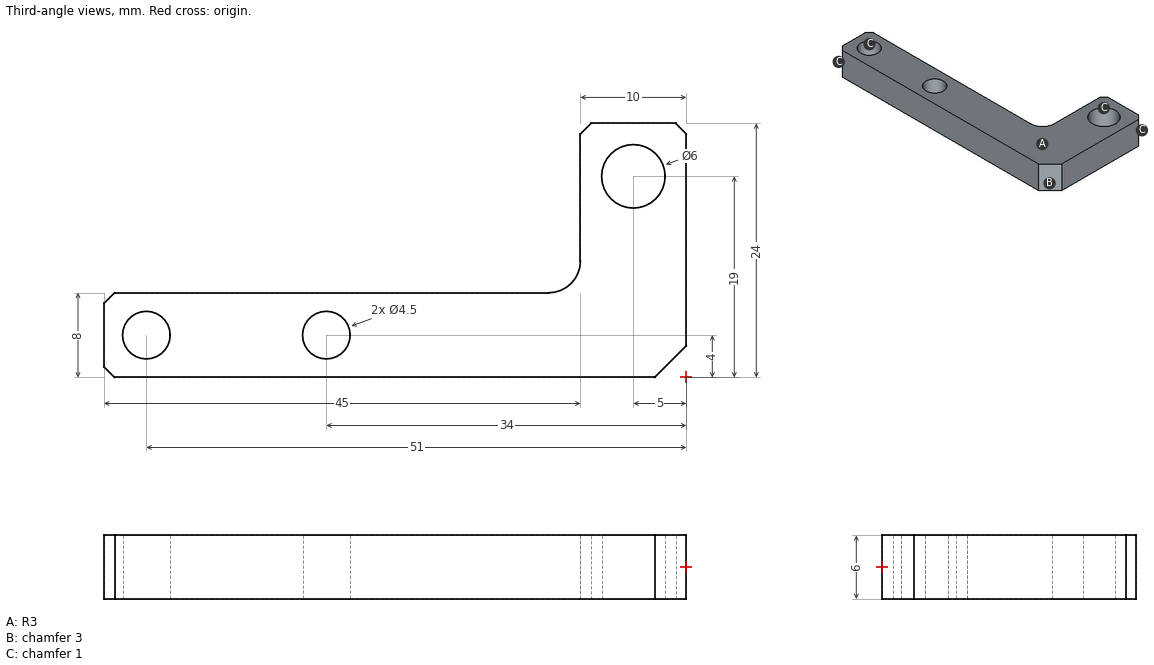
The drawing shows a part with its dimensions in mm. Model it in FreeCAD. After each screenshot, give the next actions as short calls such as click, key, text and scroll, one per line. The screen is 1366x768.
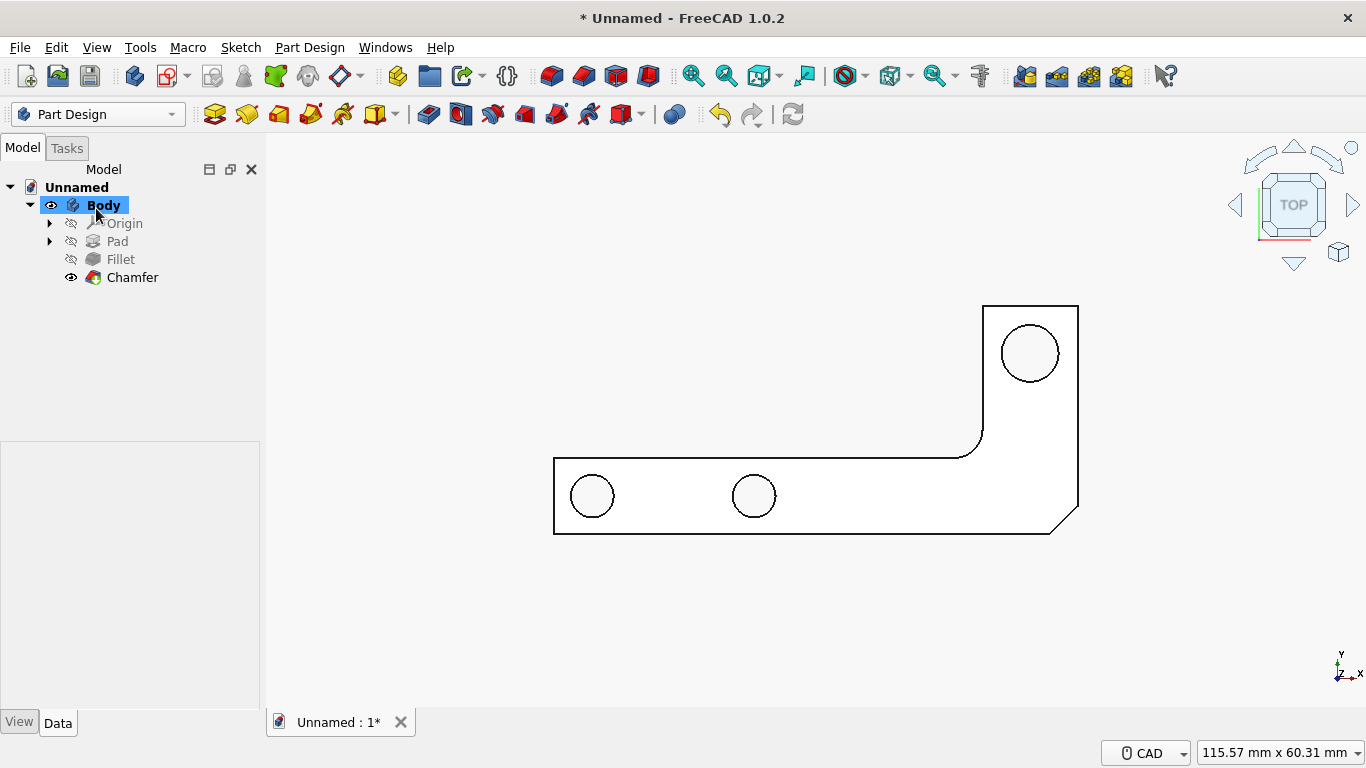
key(0)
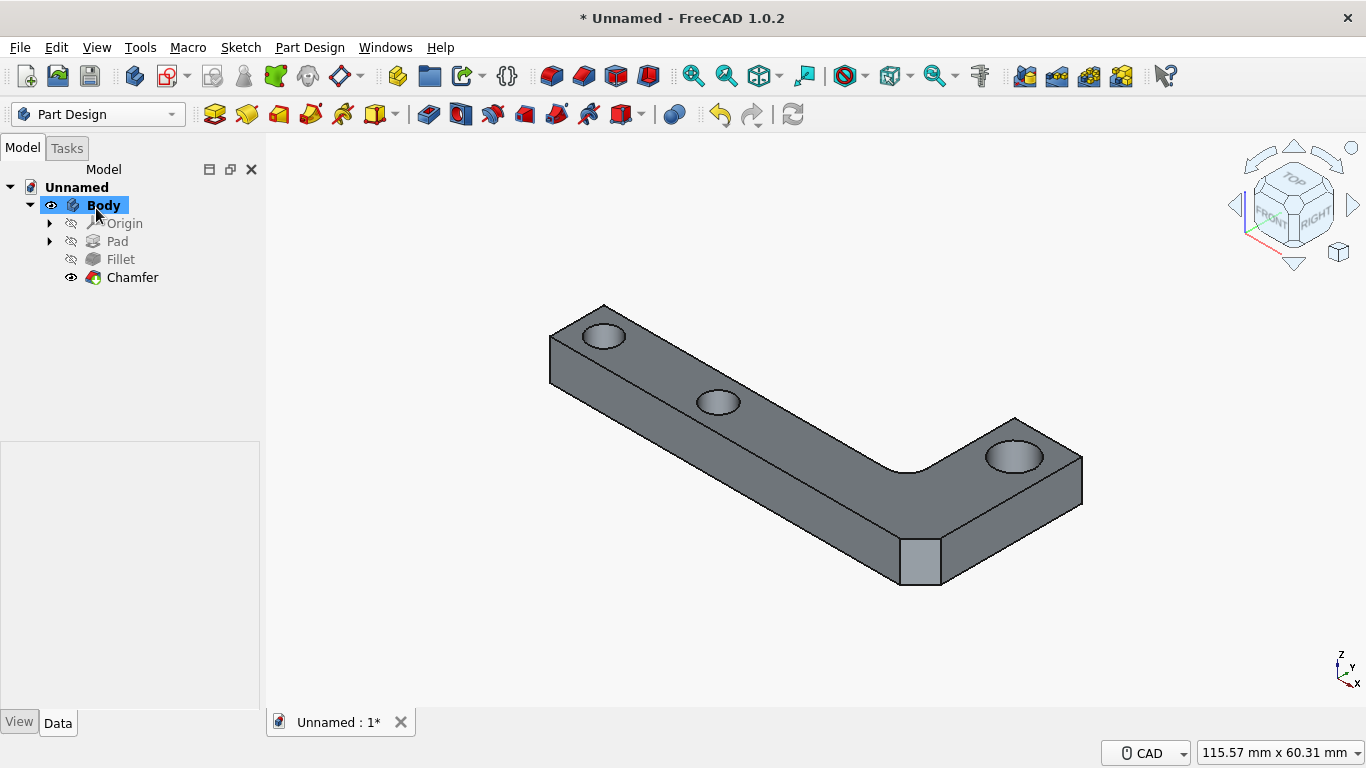
key(1)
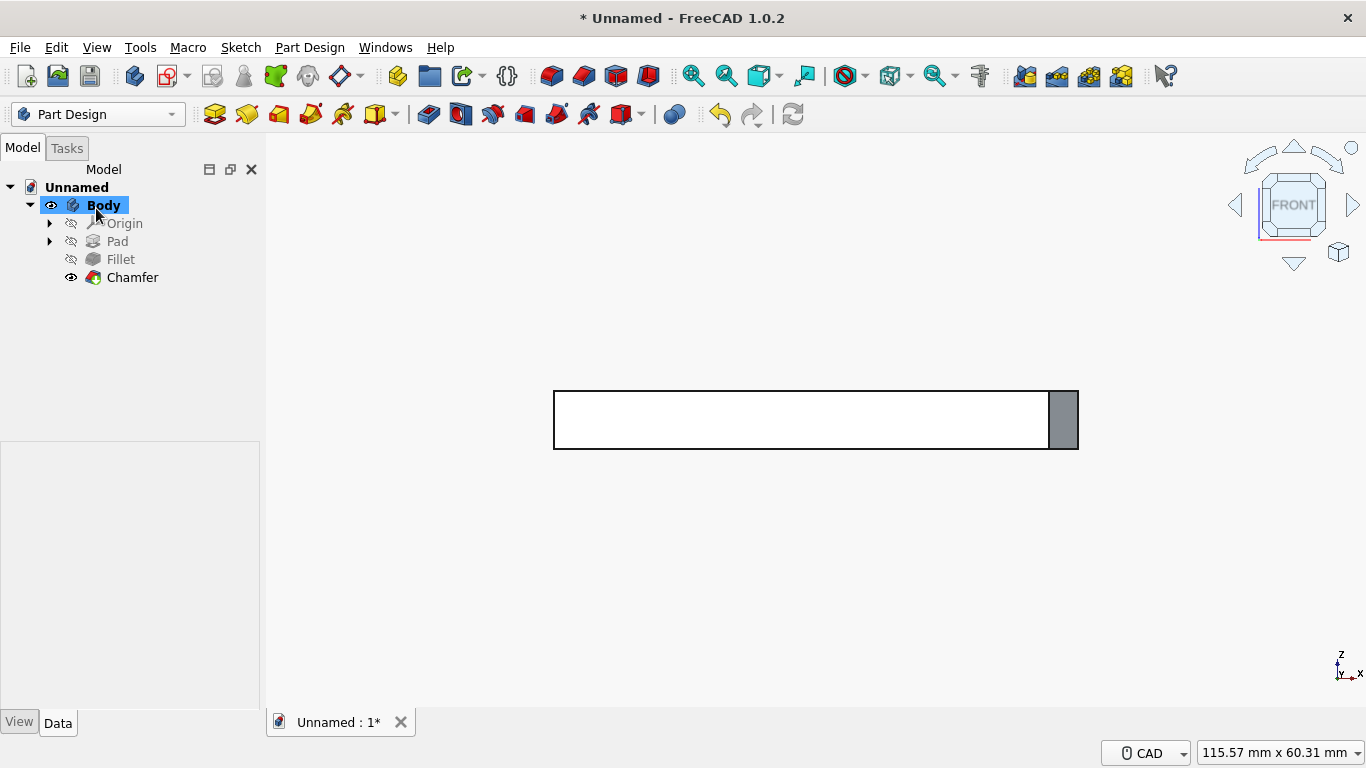
click(554, 419)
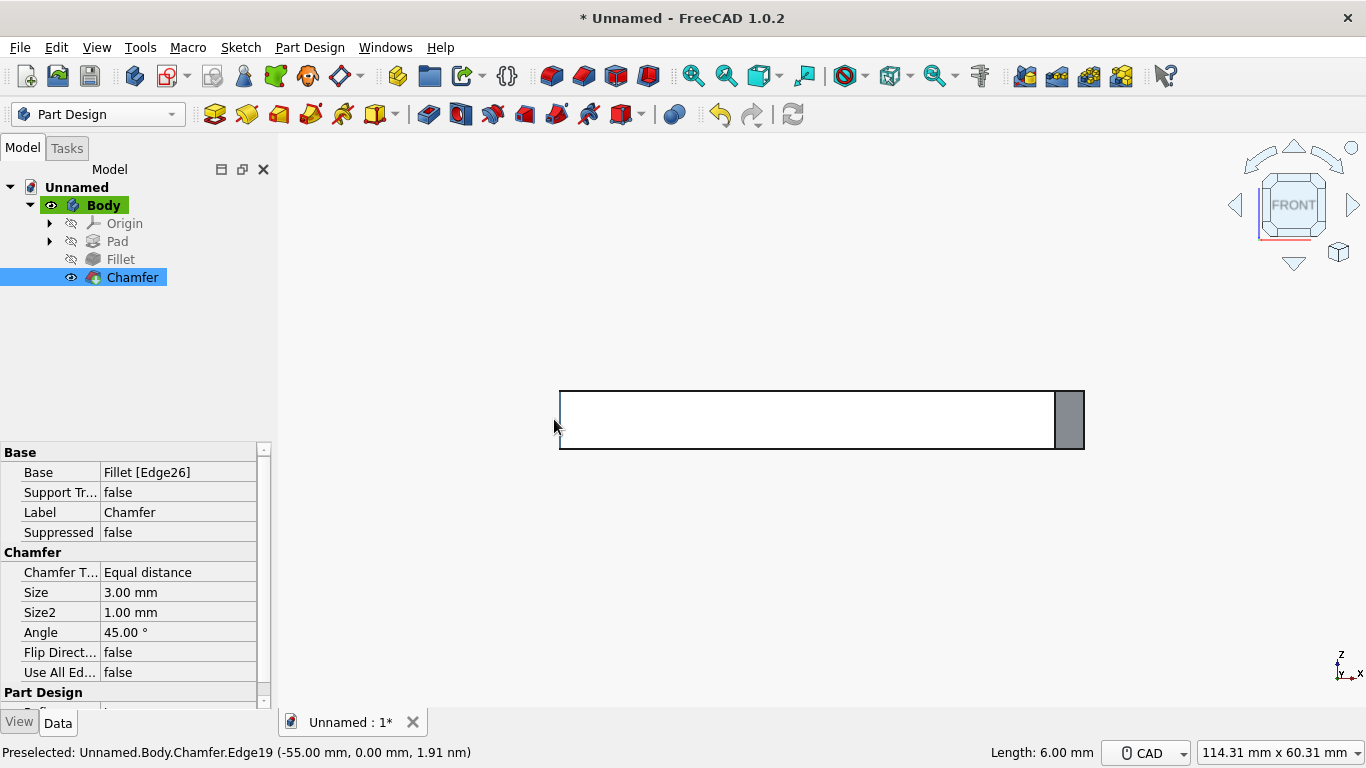
key(3)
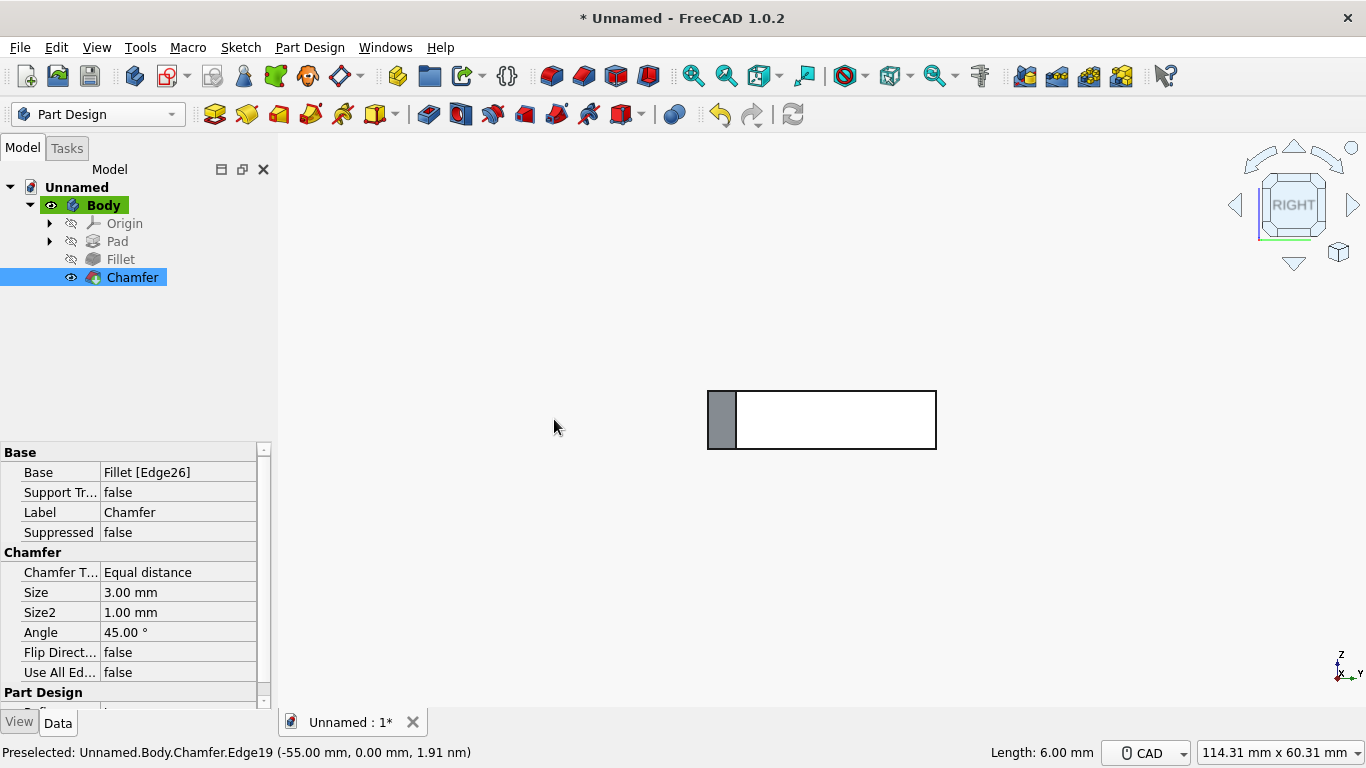
click(694, 76)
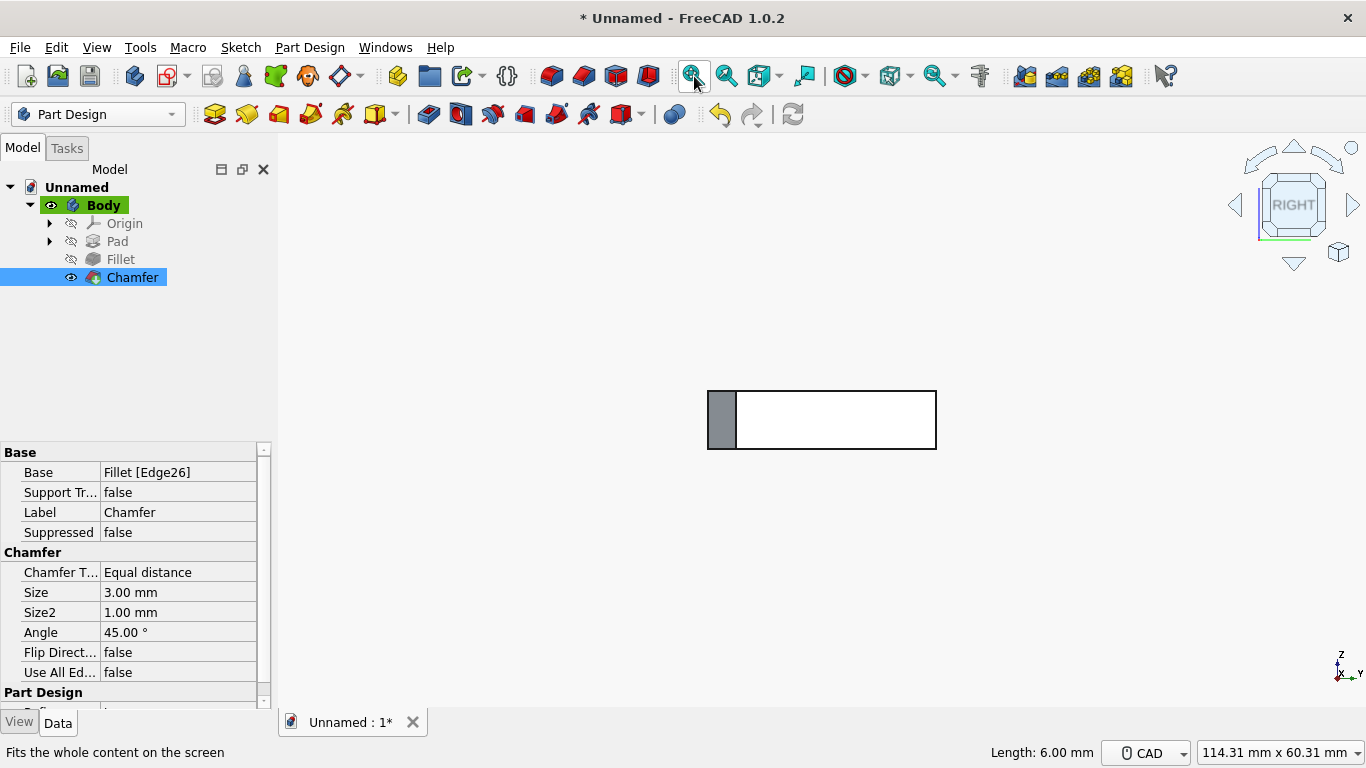
key(5)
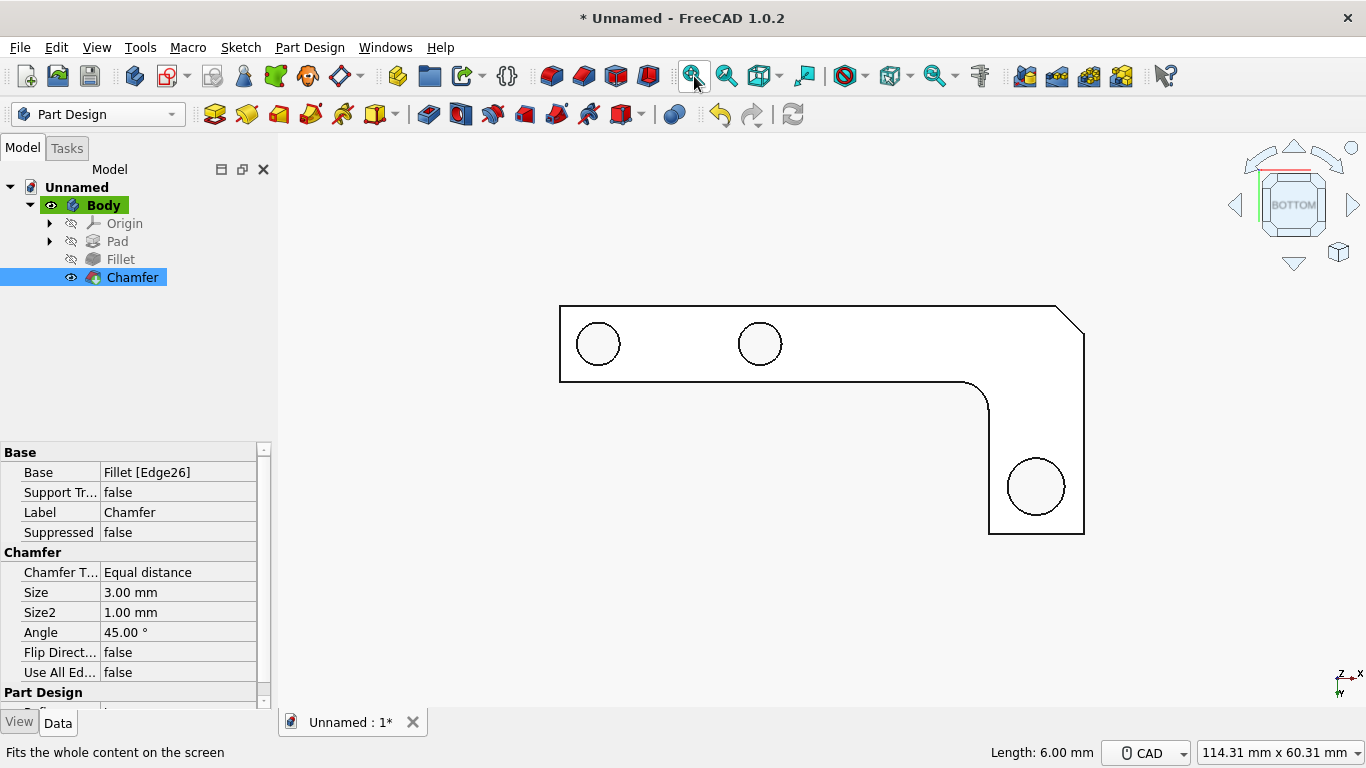
key(4)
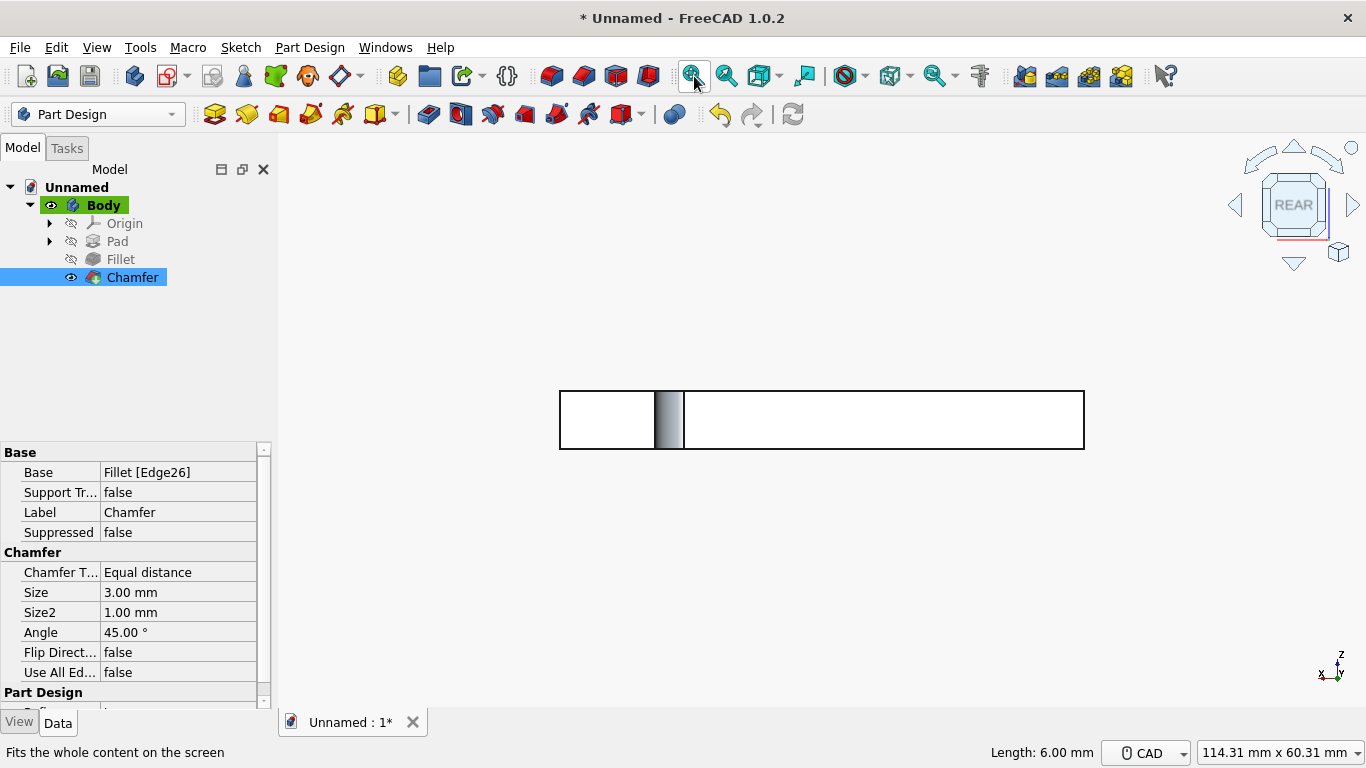
click(1084, 419, ctrl)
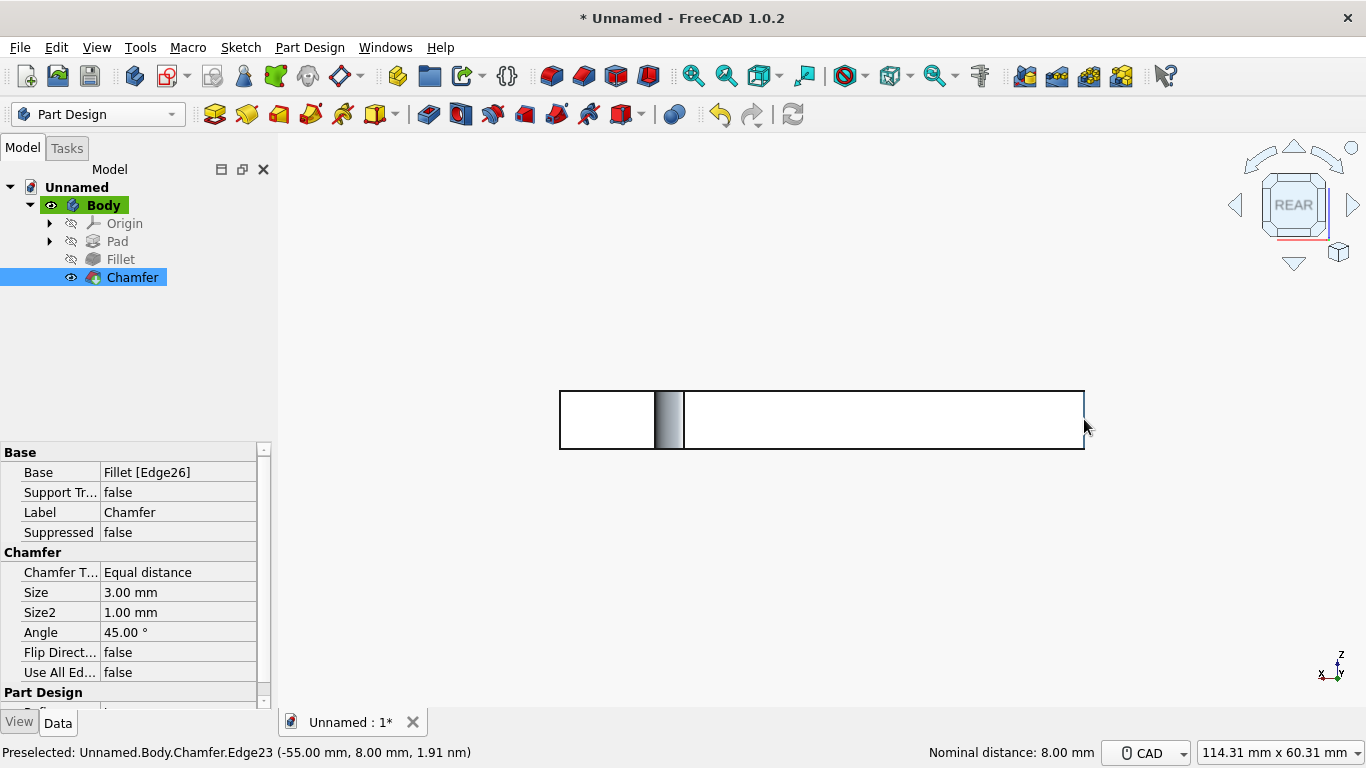
click(655, 419, ctrl)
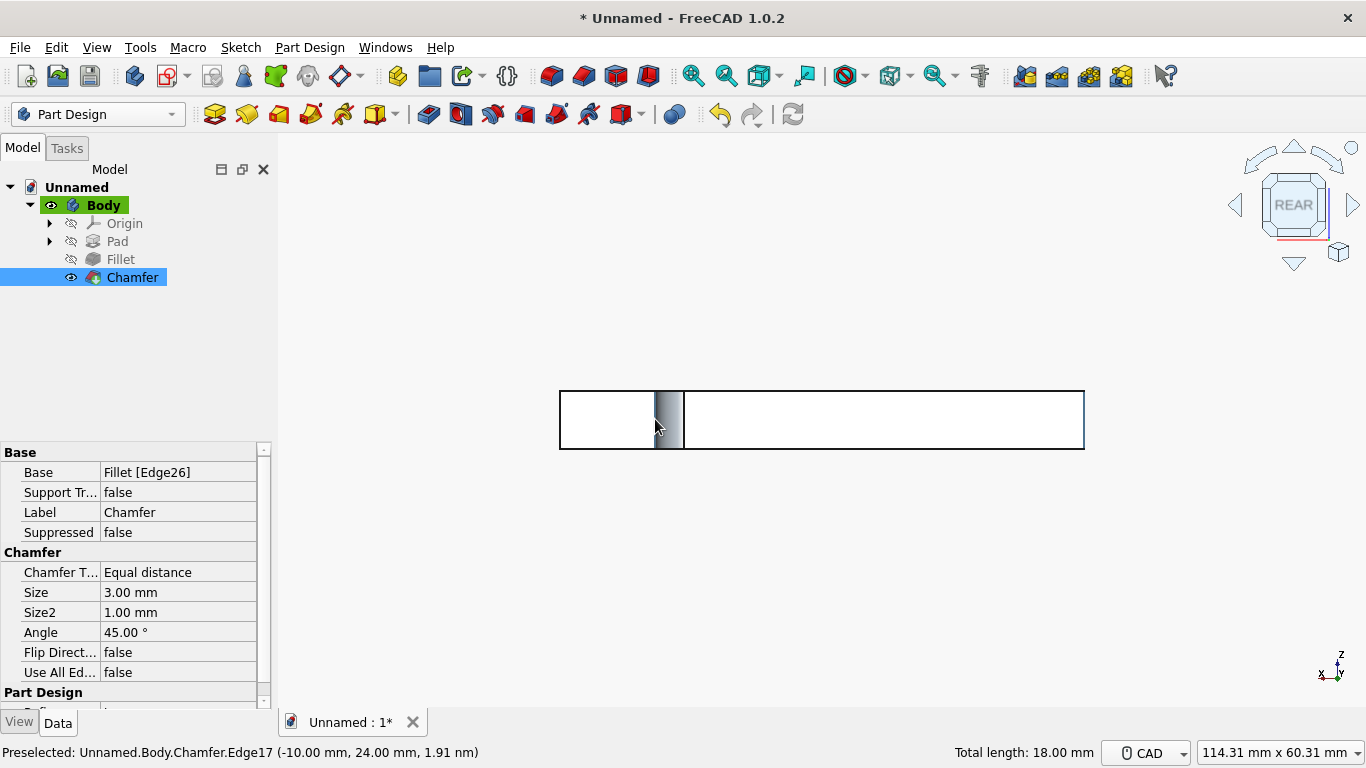
click(560, 419, ctrl)